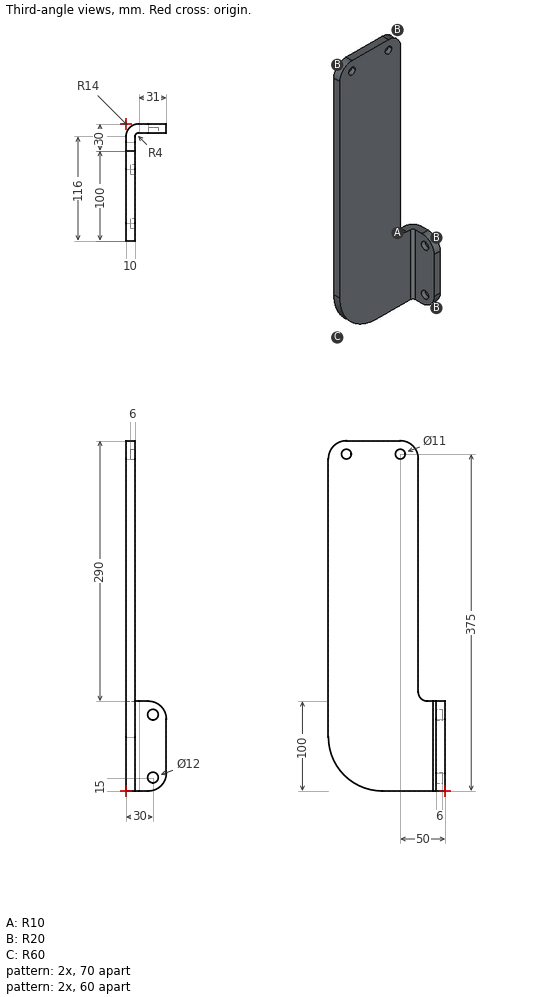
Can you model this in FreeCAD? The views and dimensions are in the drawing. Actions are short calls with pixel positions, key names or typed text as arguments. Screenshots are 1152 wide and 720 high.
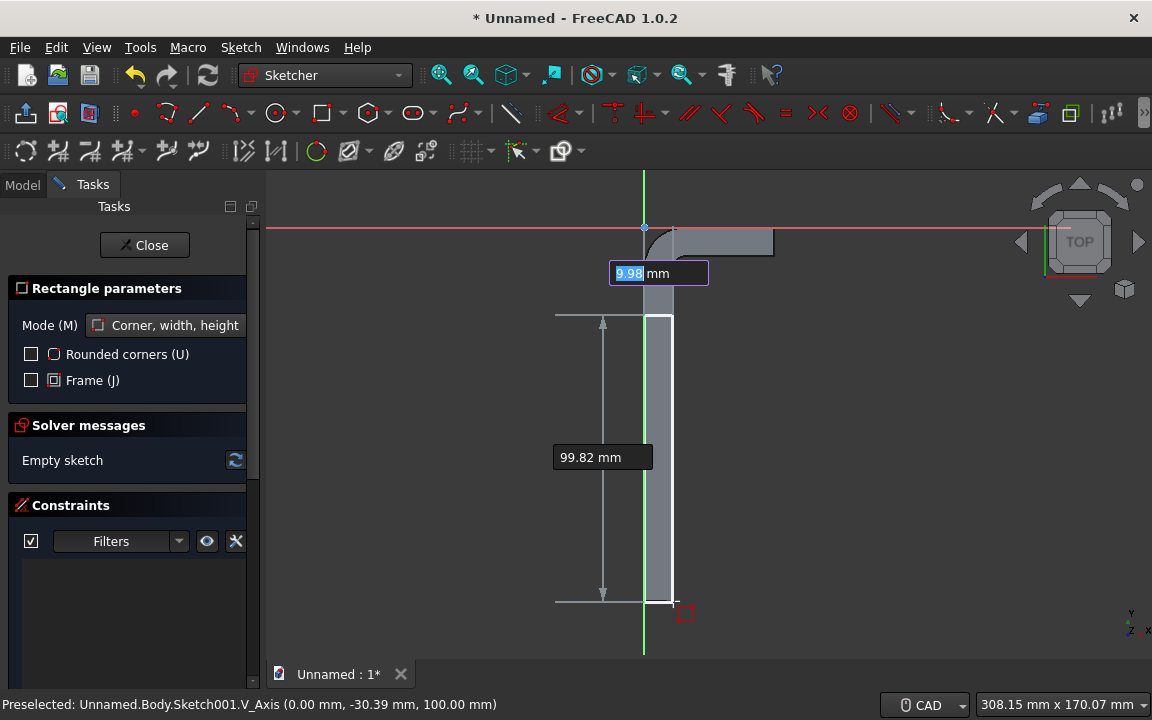
text(10)
key(Tab)
text(100)
key(Return)
key(Escape)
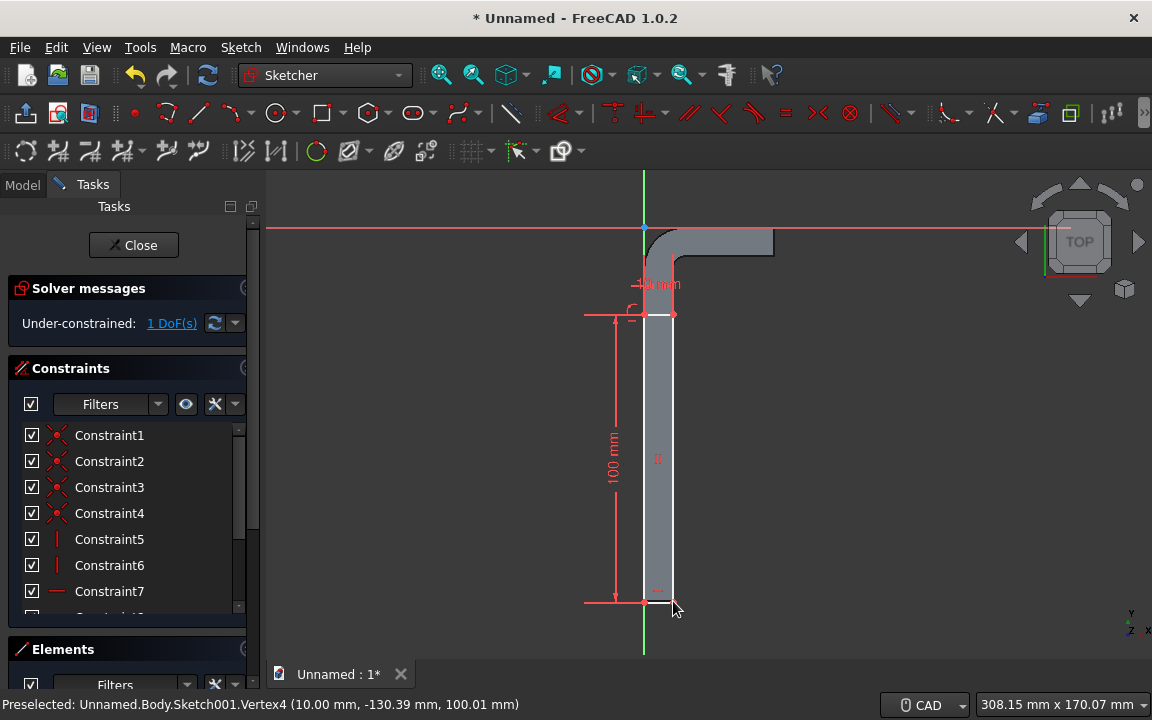
click(558, 114)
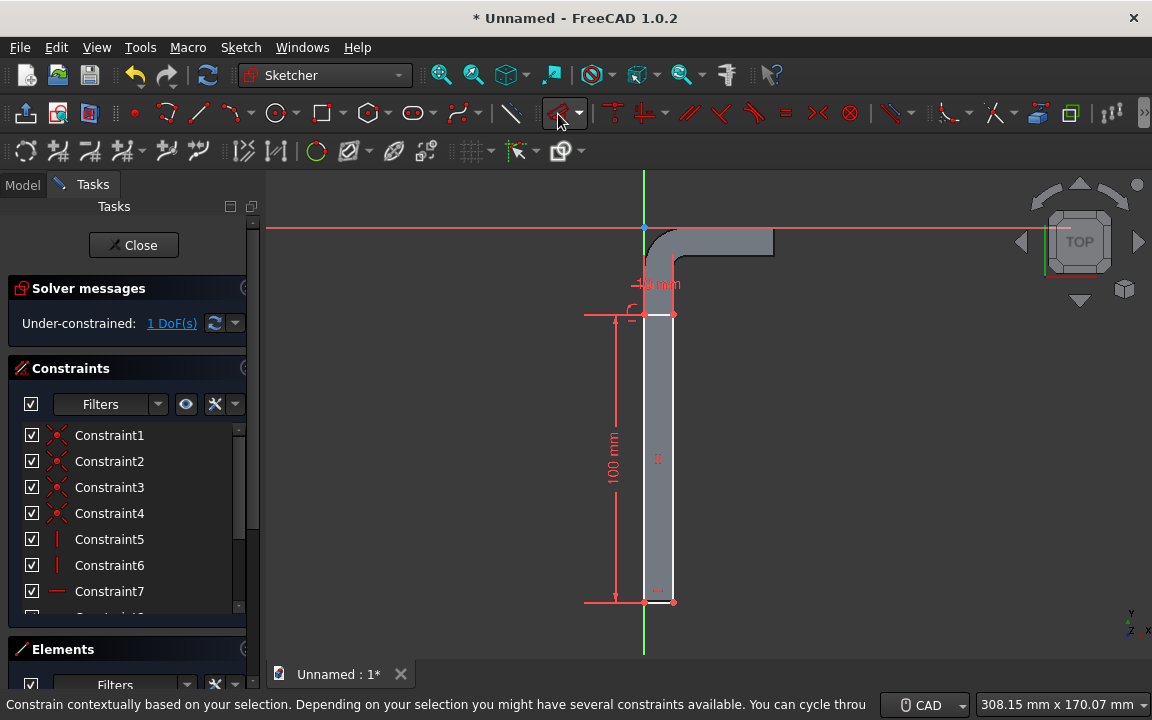
click(644, 315)
click(610, 271)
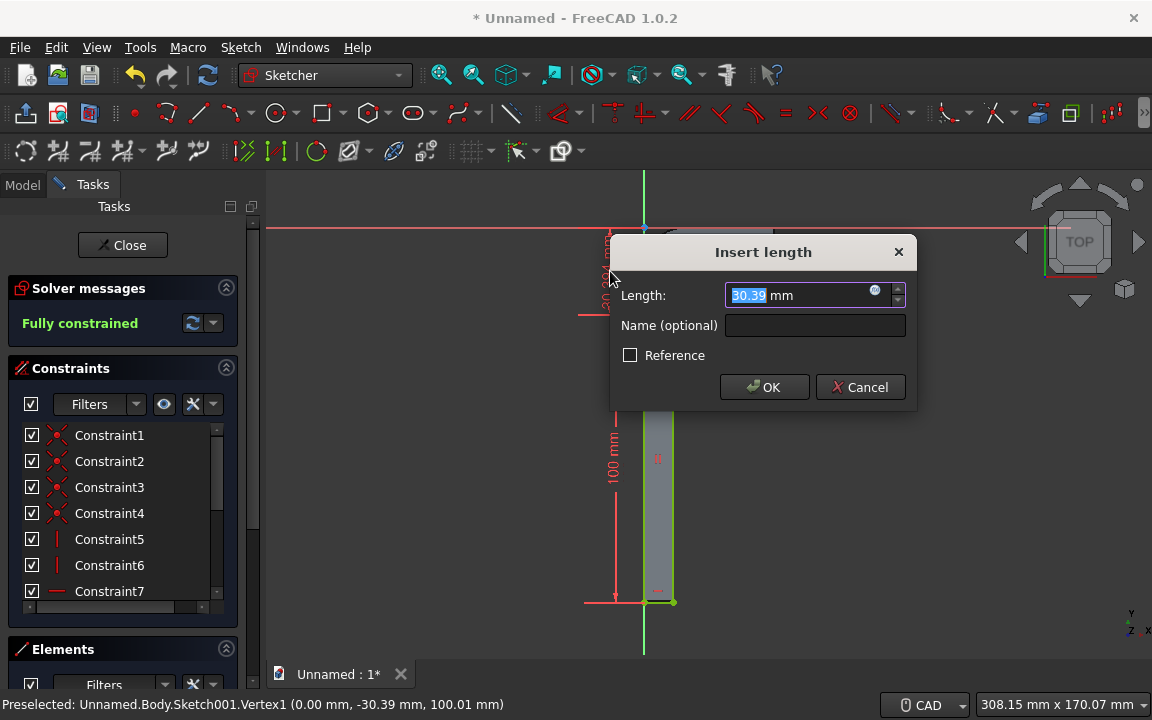
text(30)
key(Return)
key(Escape)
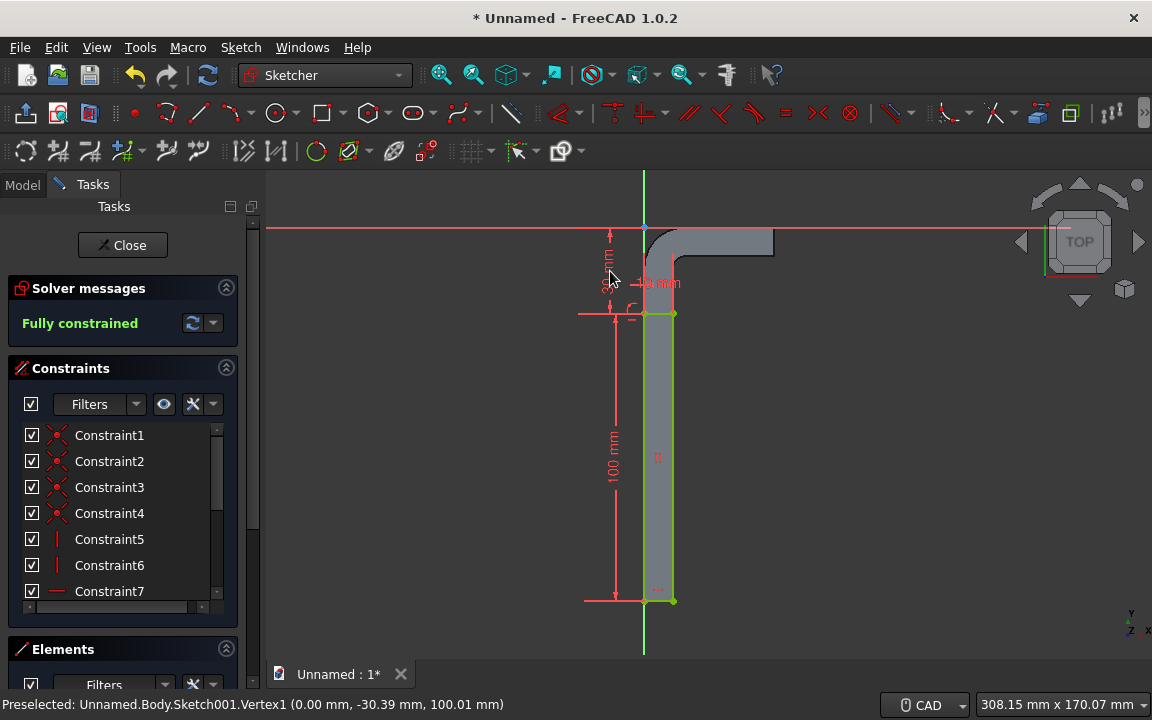
click(123, 245)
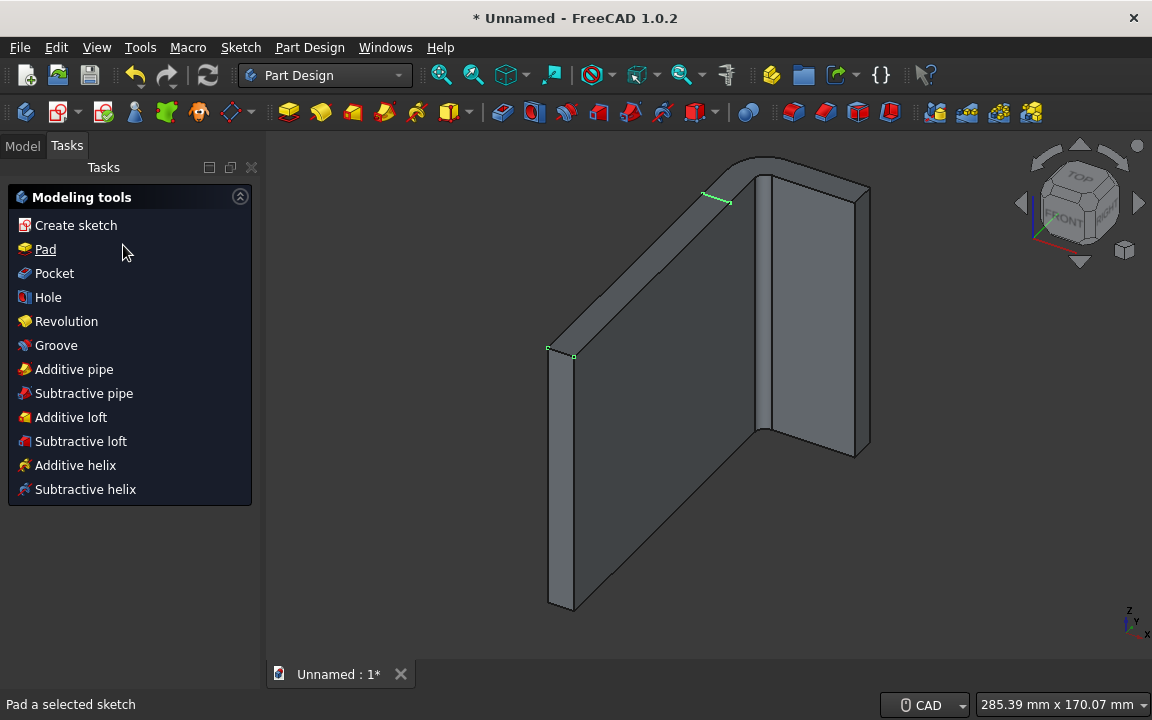
click(290, 112)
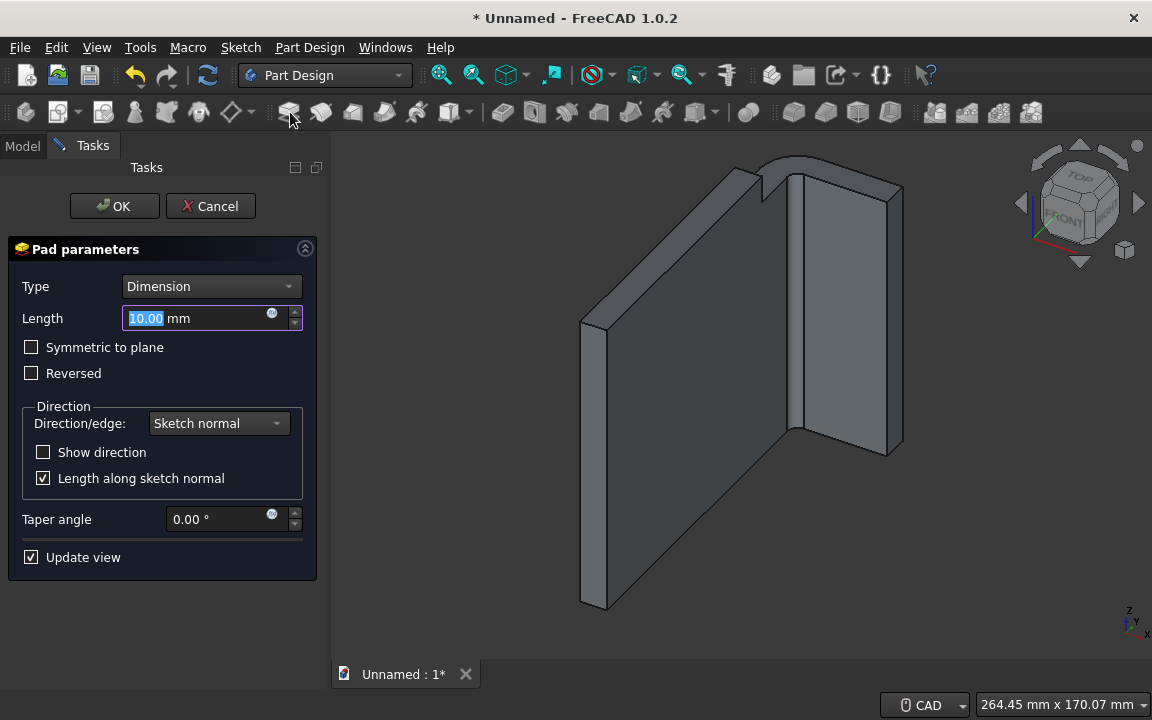
text(290)
key(Tab)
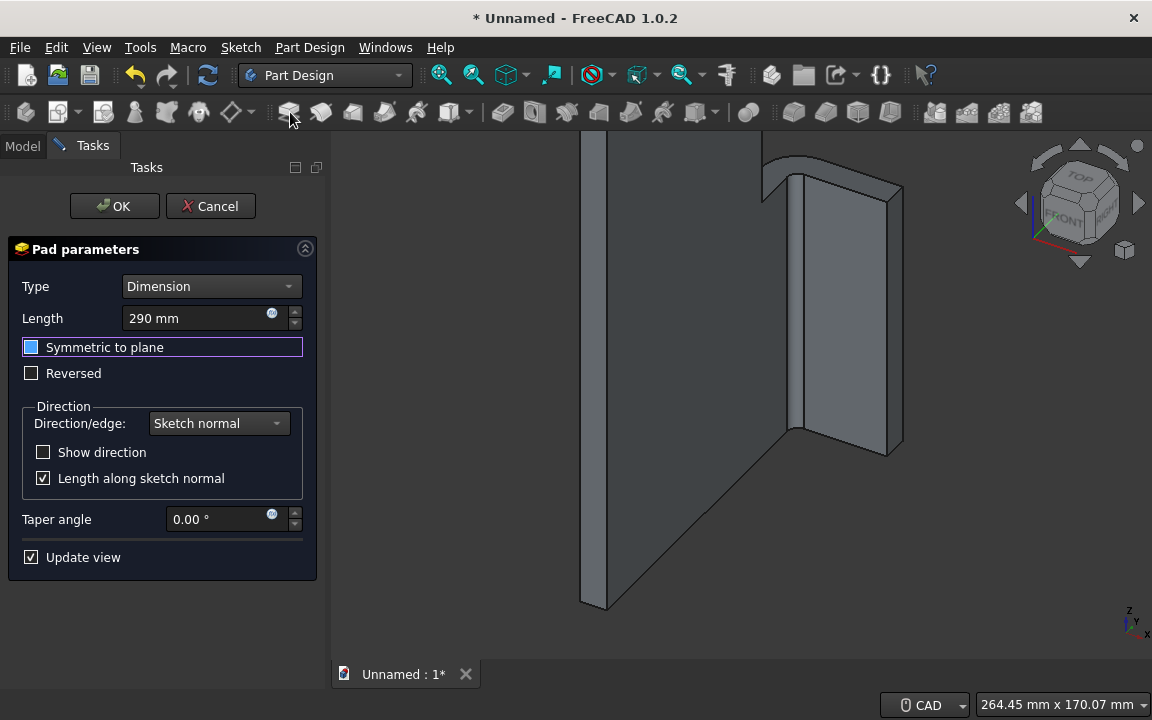
click(115, 206)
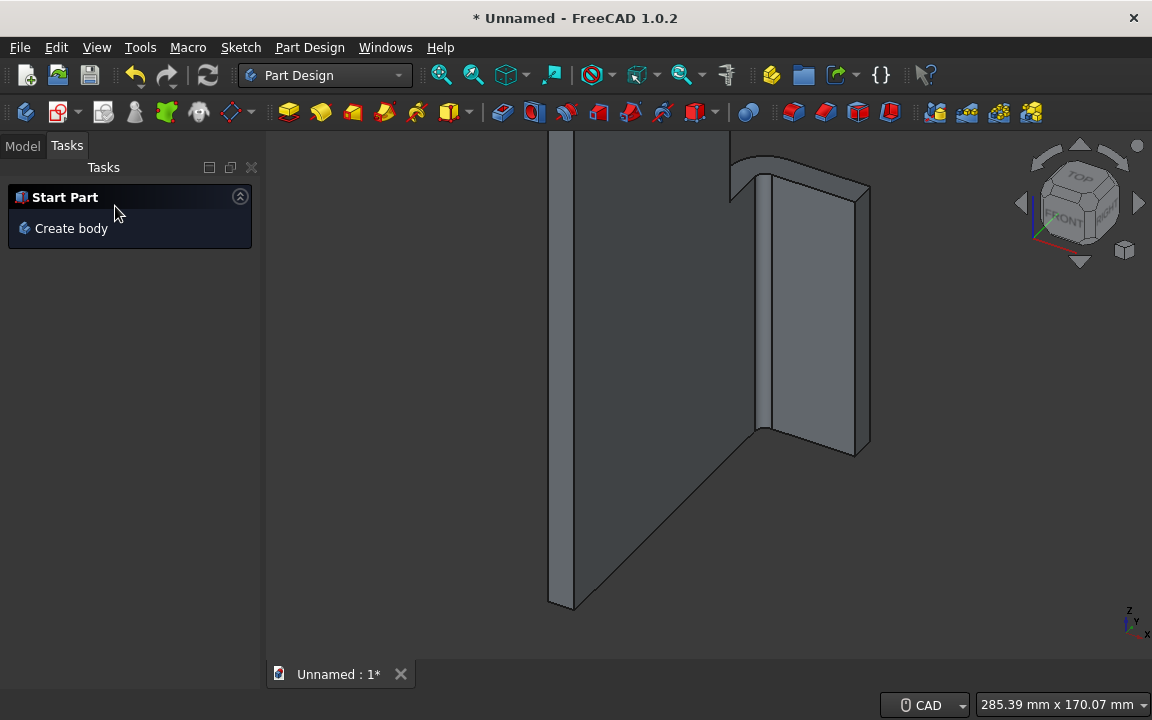
click(442, 76)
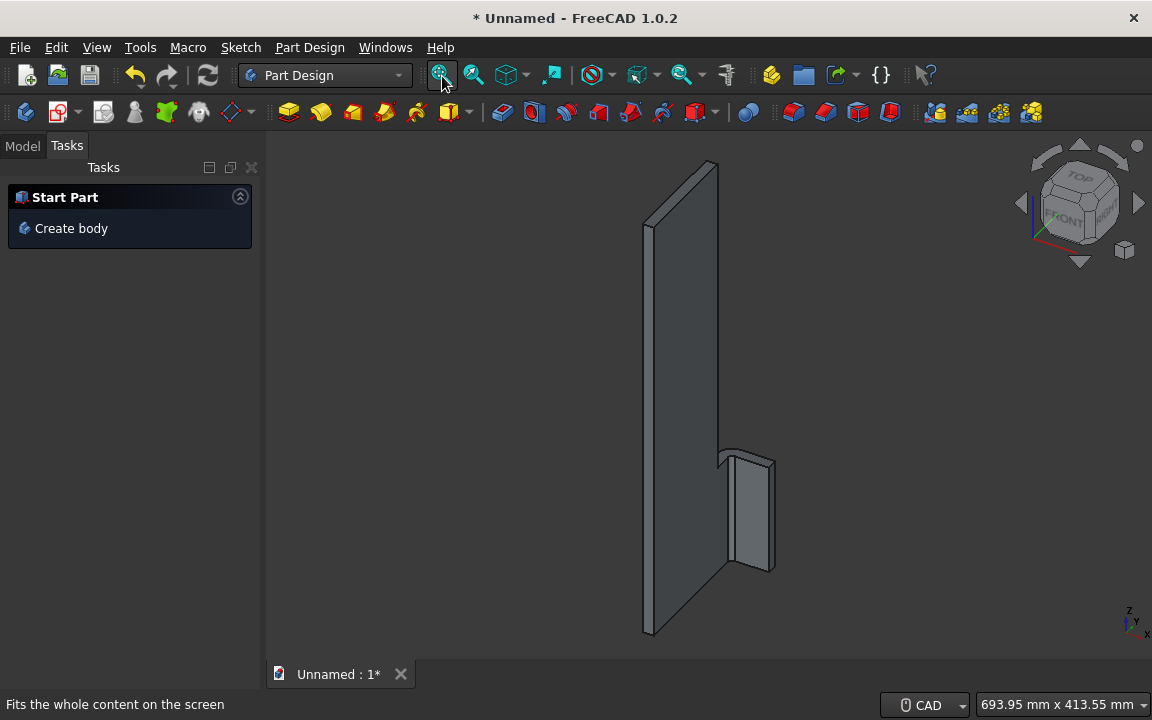
scroll(712, 465, up, 6)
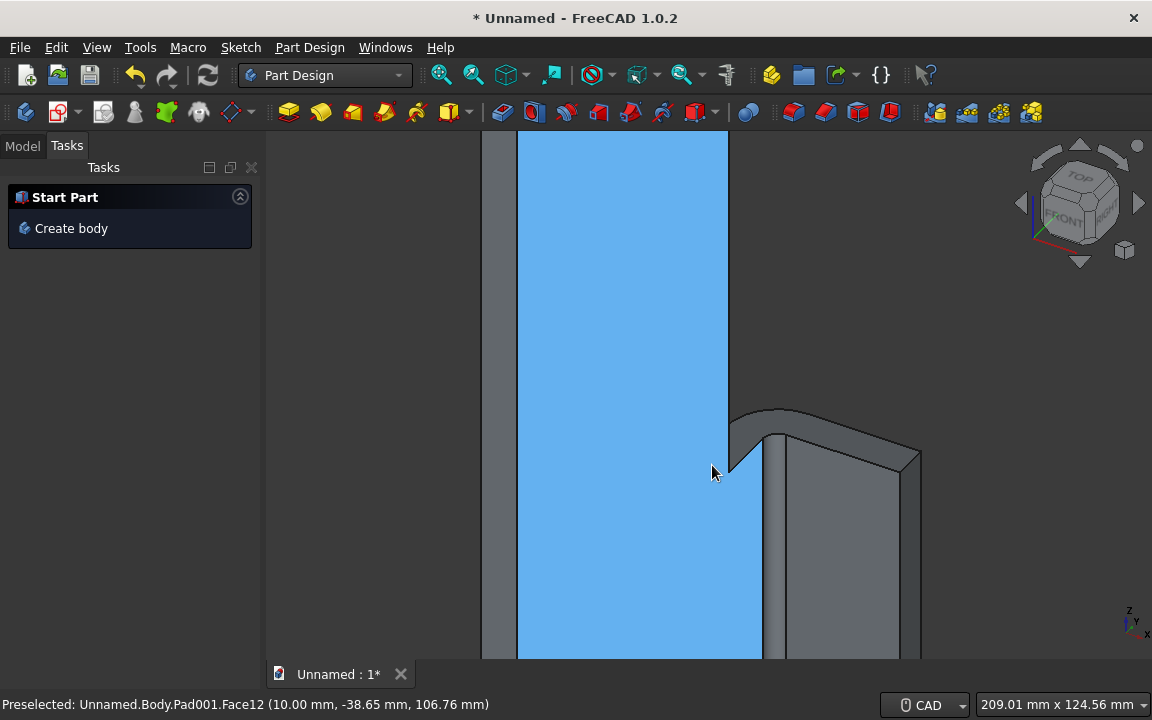
click(442, 76)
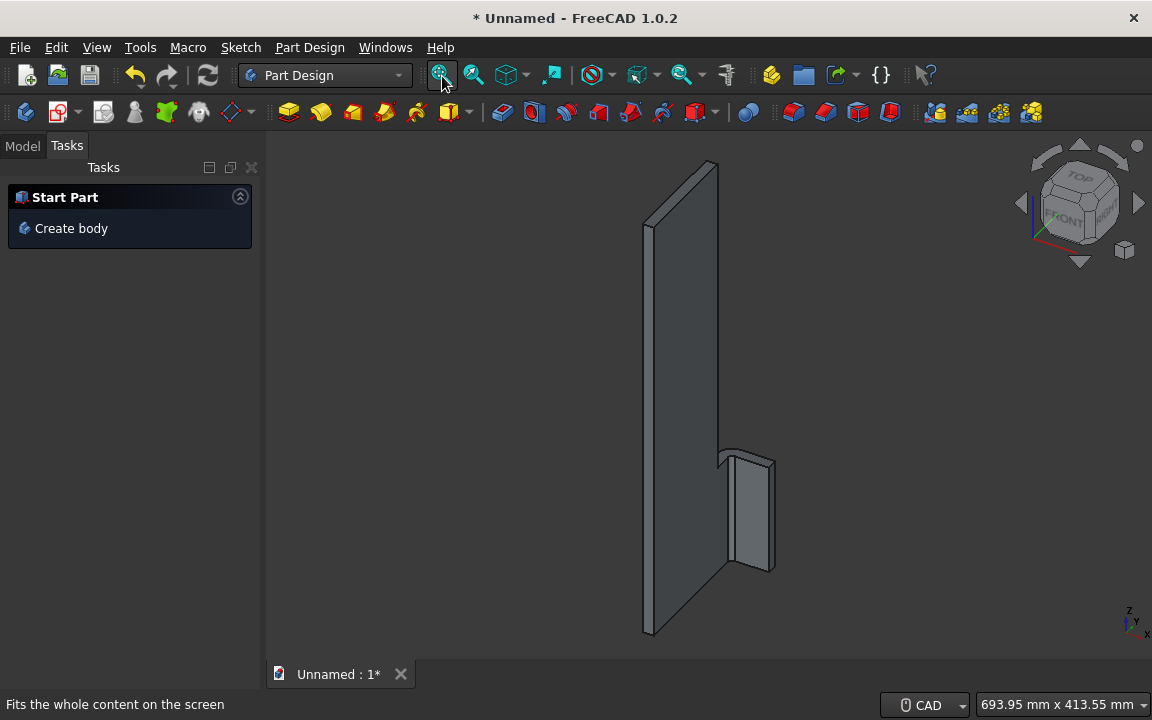
key(0)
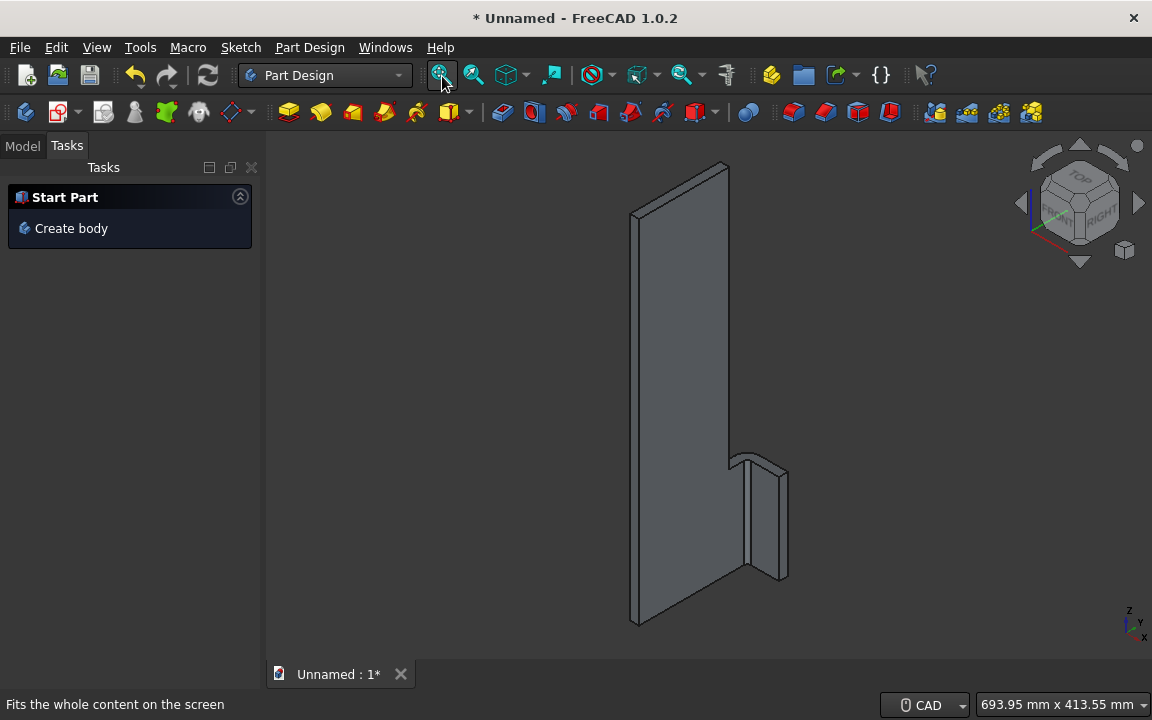
scroll(725, 466, up, 6)